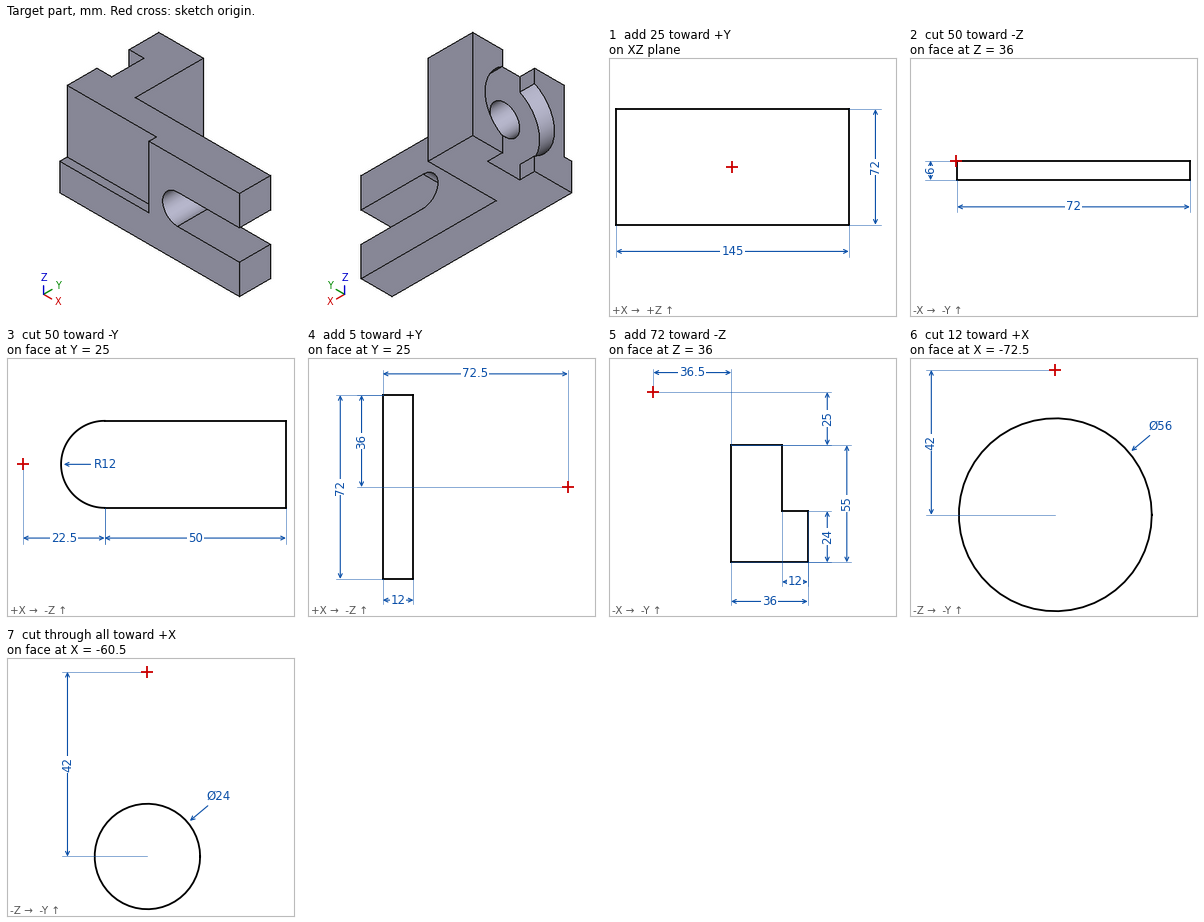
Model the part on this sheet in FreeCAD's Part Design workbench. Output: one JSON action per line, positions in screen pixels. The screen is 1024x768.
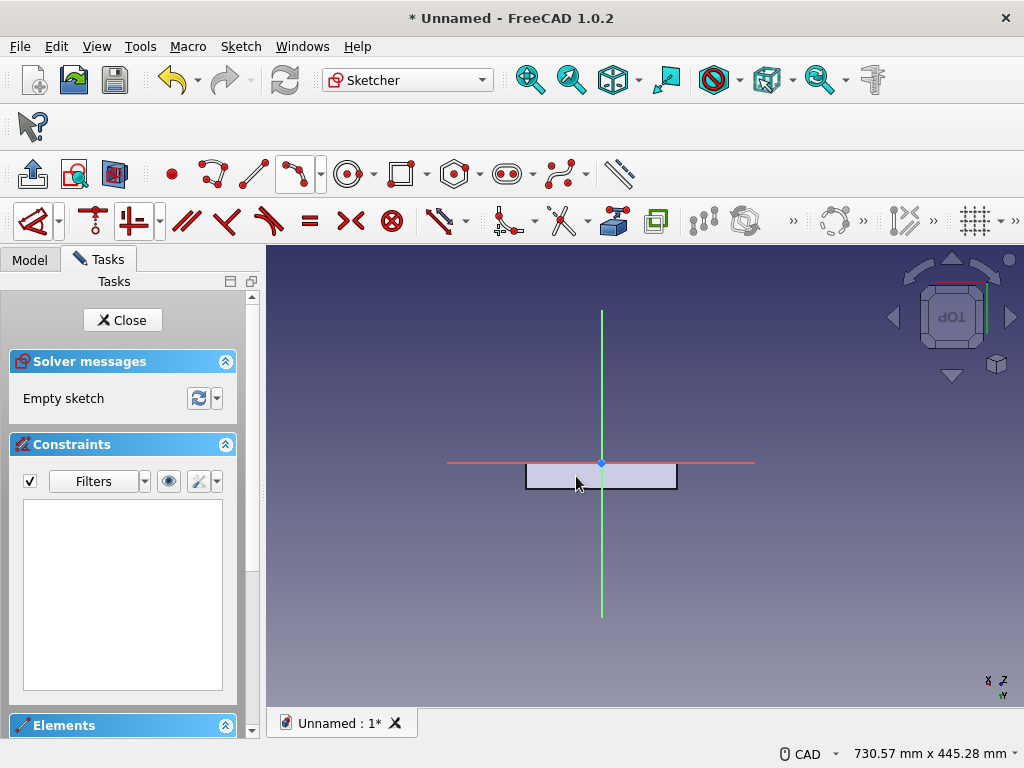
{"action": "scroll", "coordinate": [655, 464], "scroll_direction": "up", "scroll_amount": 8}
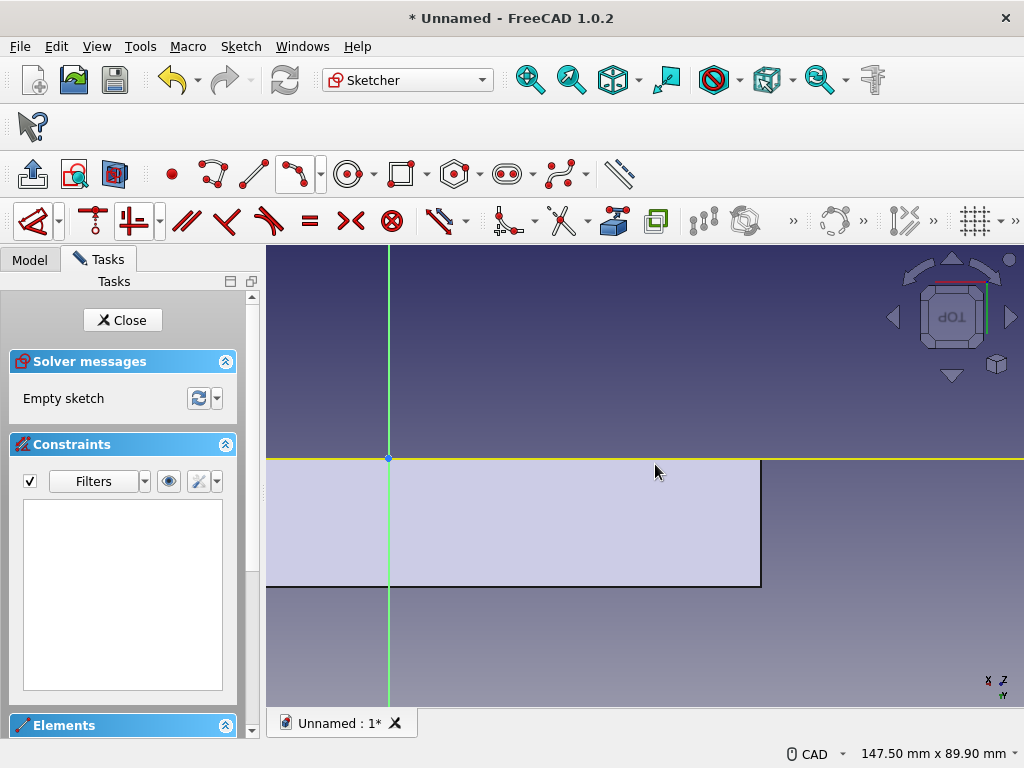
{"action": "left_click", "coordinate": [400, 174]}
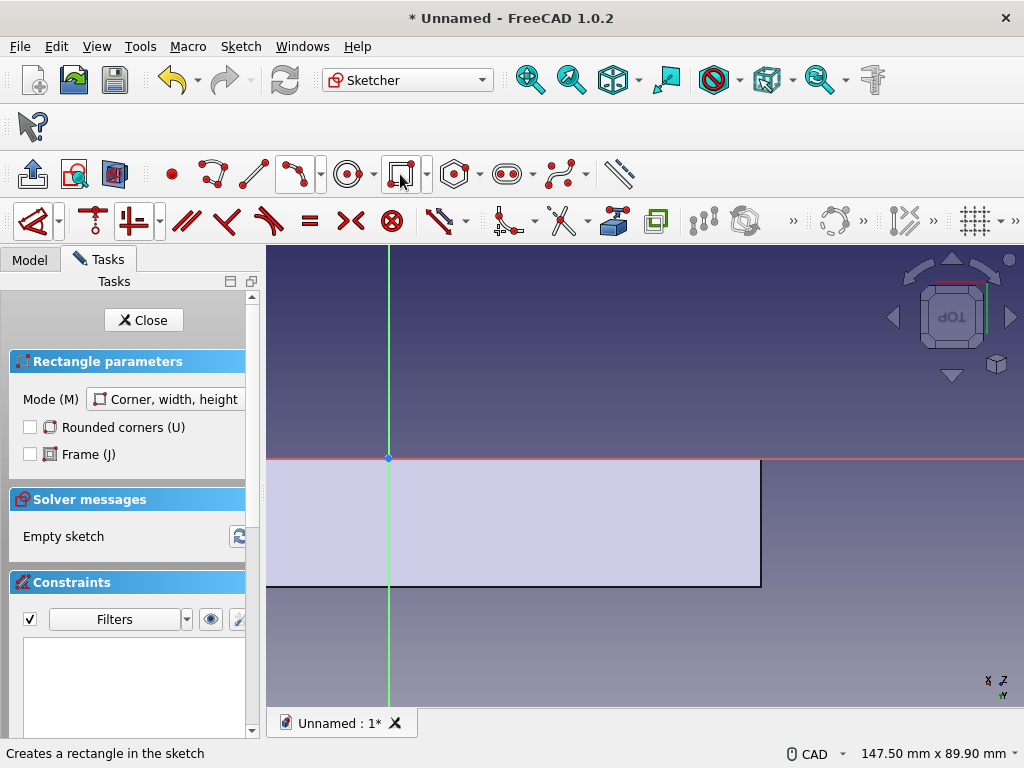
{"action": "scroll", "coordinate": [391, 459], "scroll_direction": "up", "scroll_amount": 10}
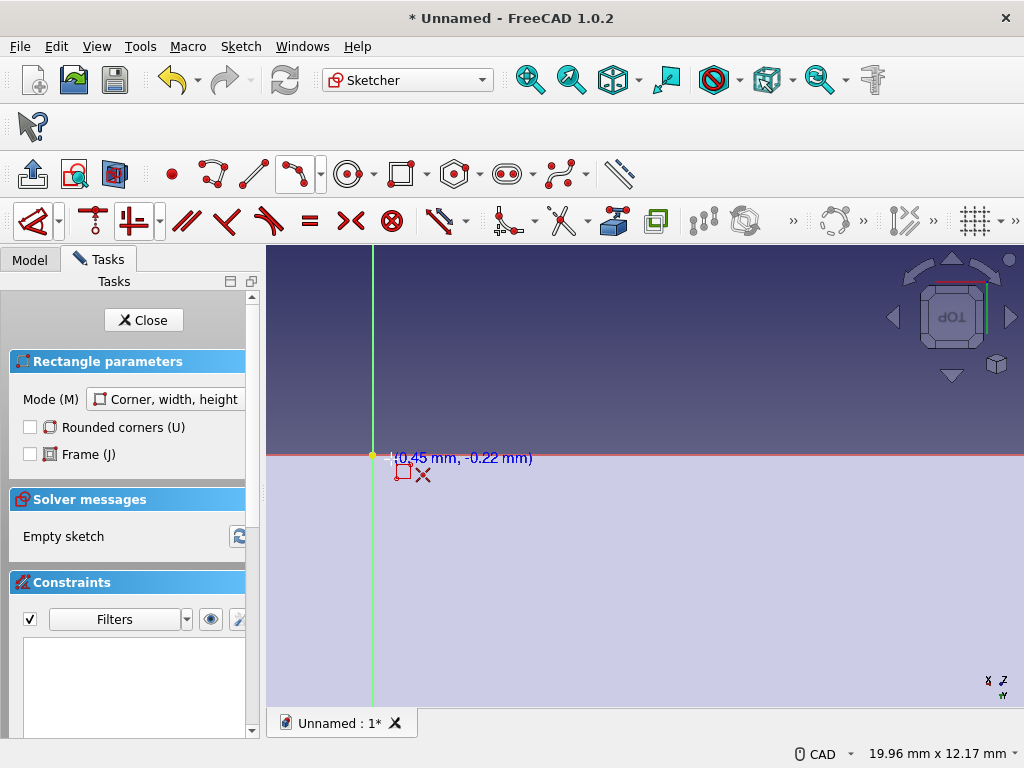
{"action": "left_click", "coordinate": [392, 455]}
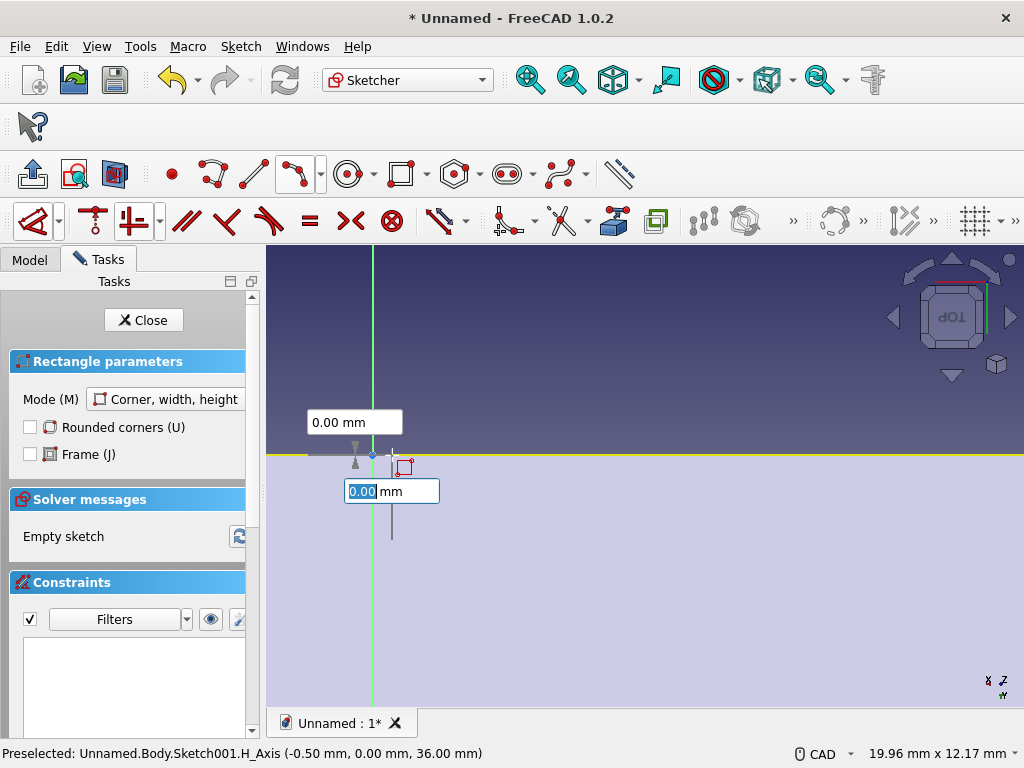
{"action": "scroll", "coordinate": [393, 461], "scroll_direction": "down", "scroll_amount": 10}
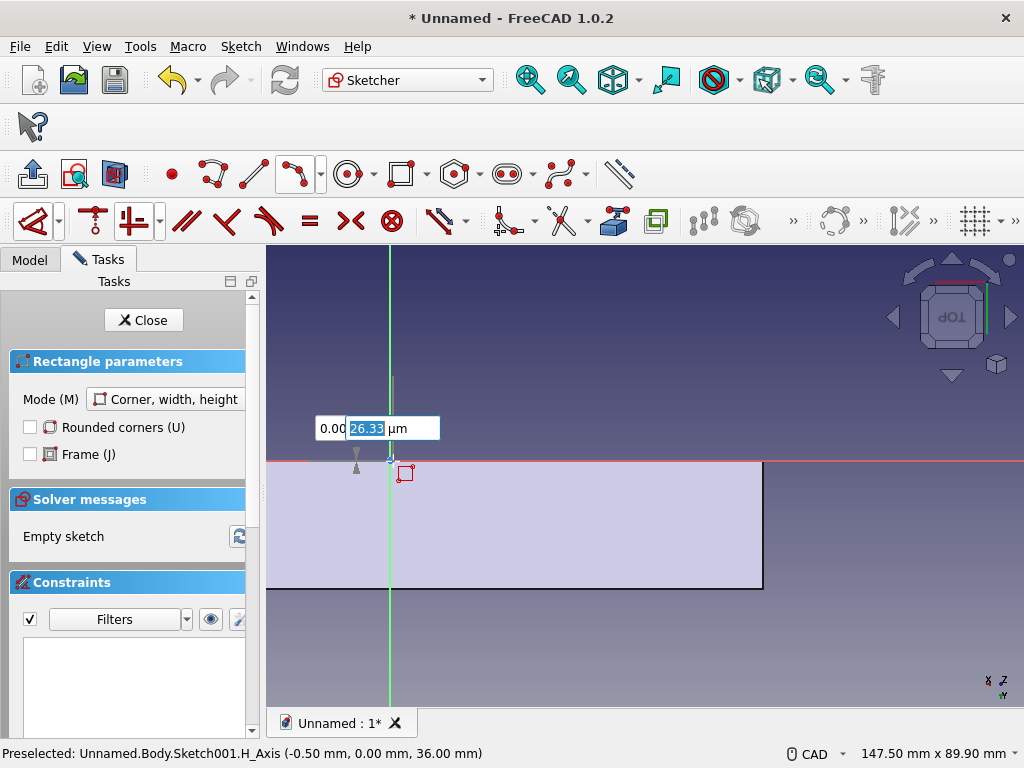
{"action": "left_click", "coordinate": [763, 491]}
{"action": "key", "text": "Escape"}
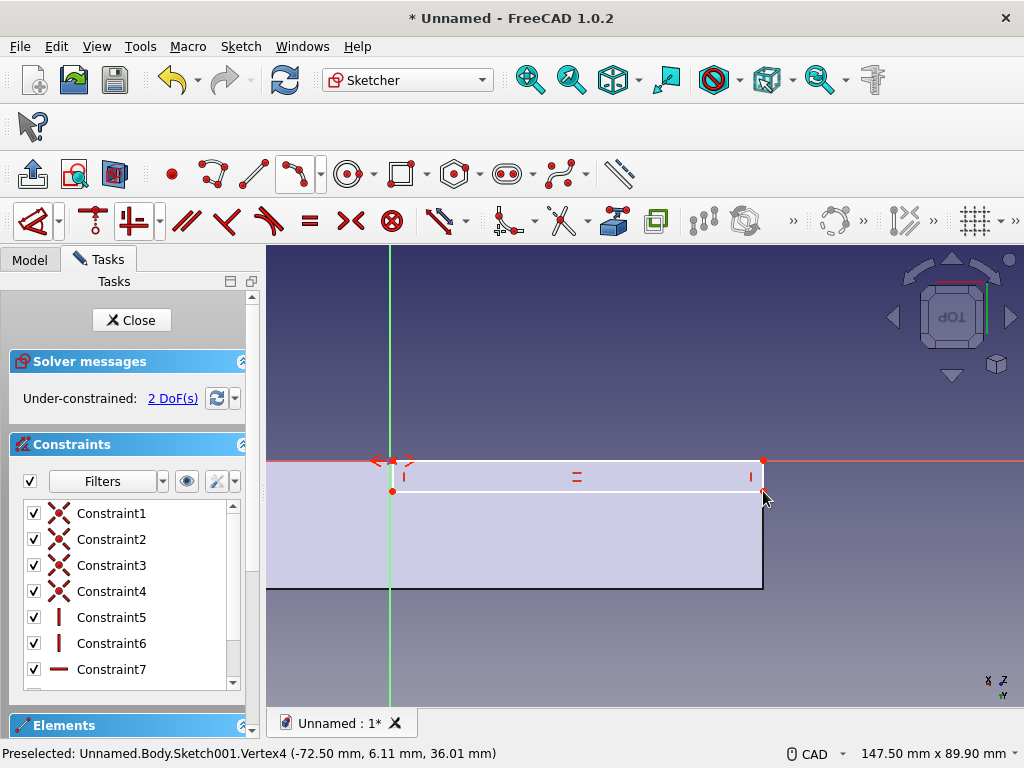
{"action": "scroll", "coordinate": [393, 470], "scroll_direction": "up", "scroll_amount": 2}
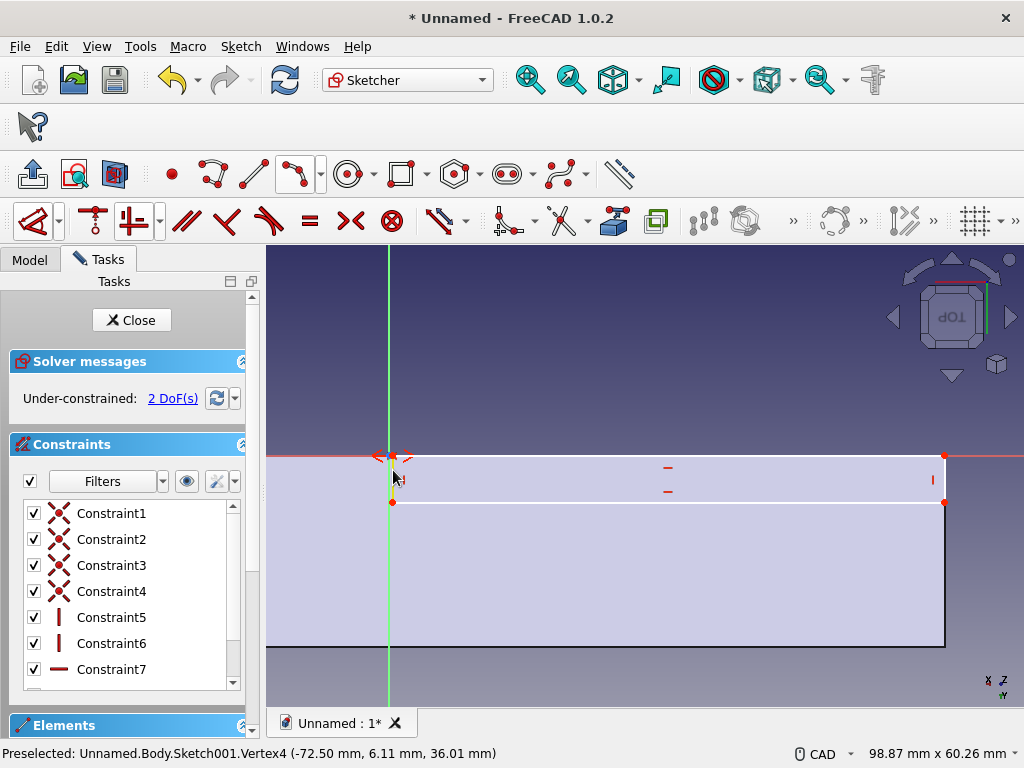
{"action": "left_click", "coordinate": [393, 470]}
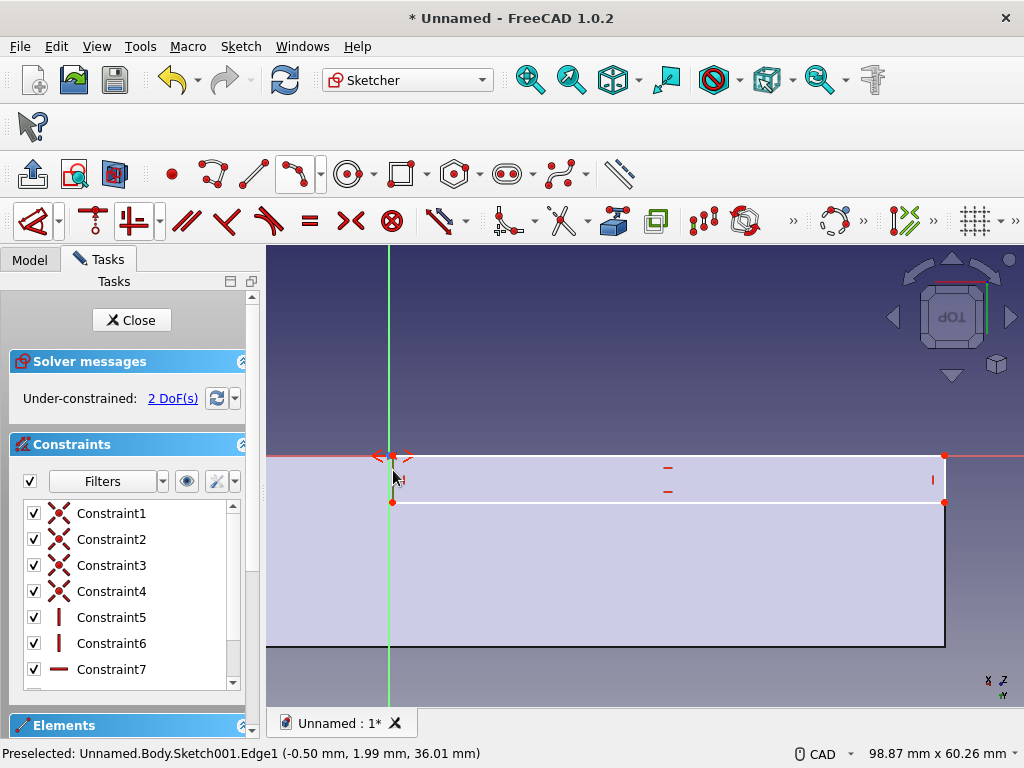
{"action": "key", "text": "i"}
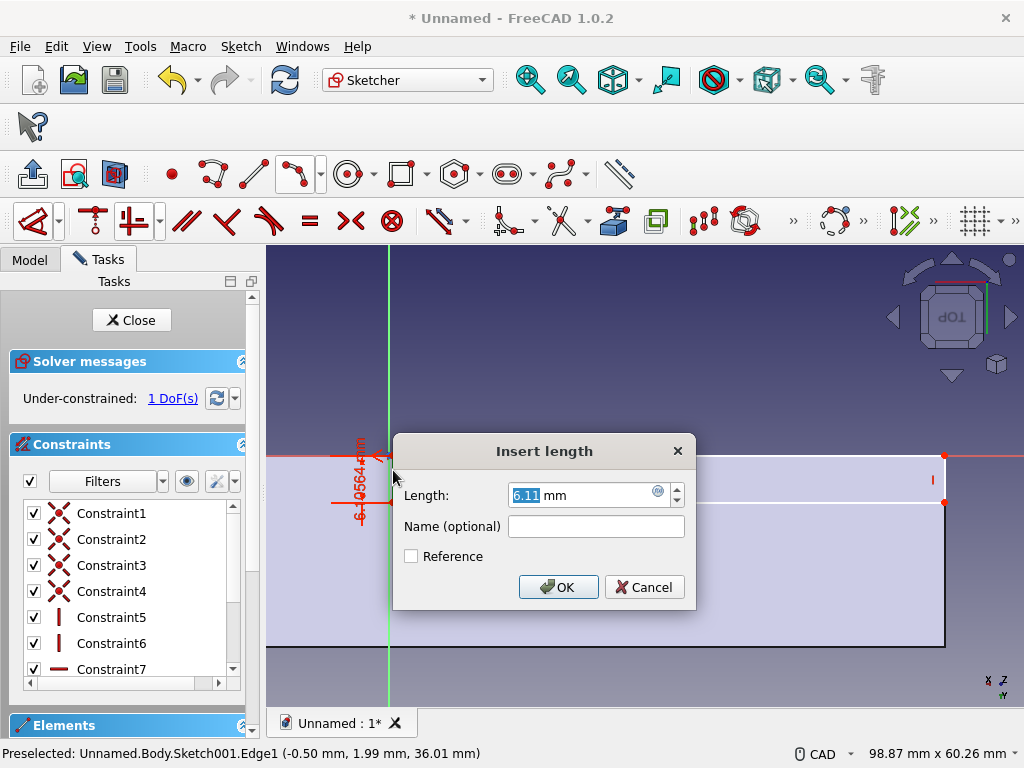
{"action": "type", "text": "6"}
{"action": "key", "text": "Return"}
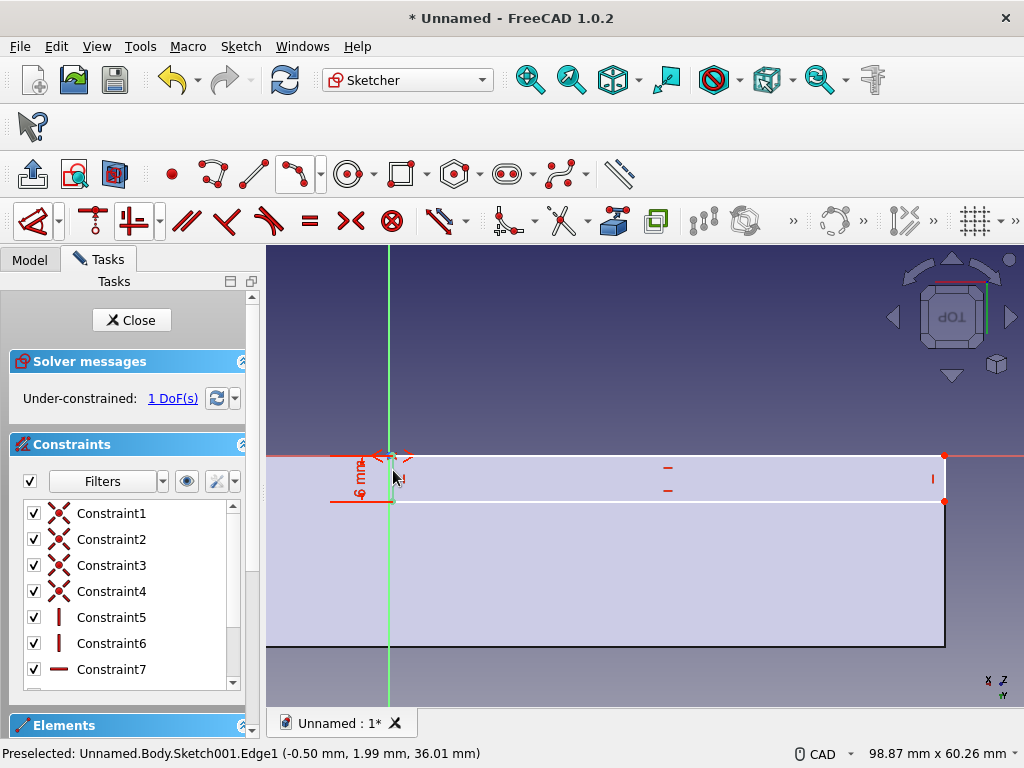
{"action": "left_click", "coordinate": [558, 502]}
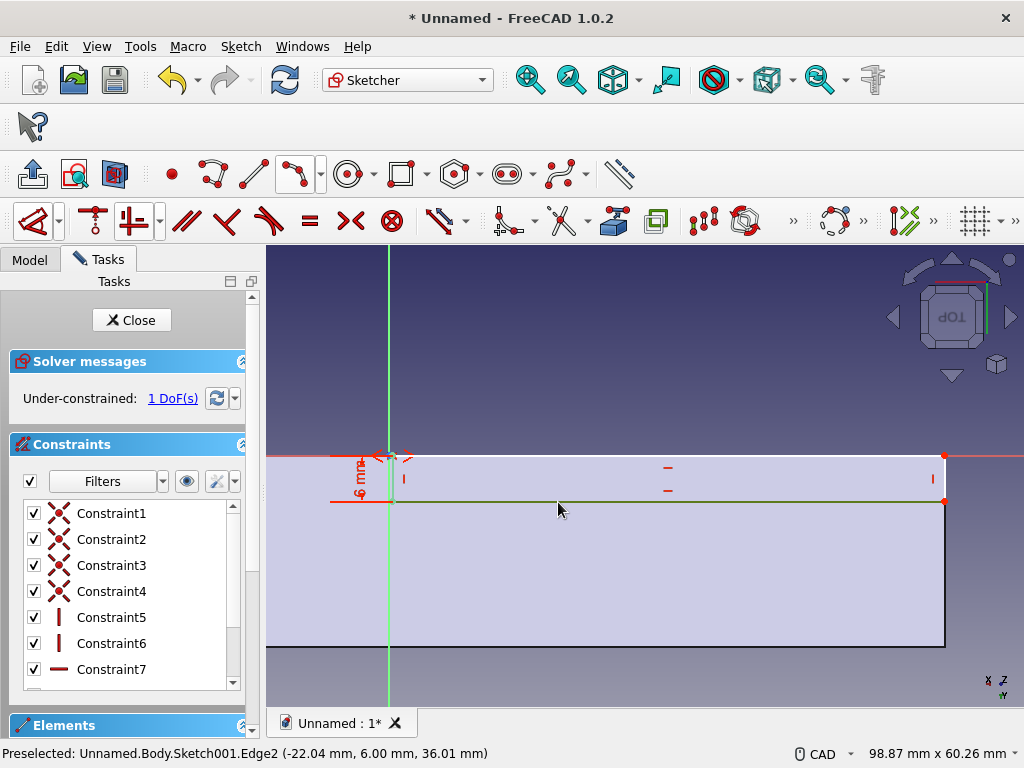
{"action": "left_click", "coordinate": [58, 222]}